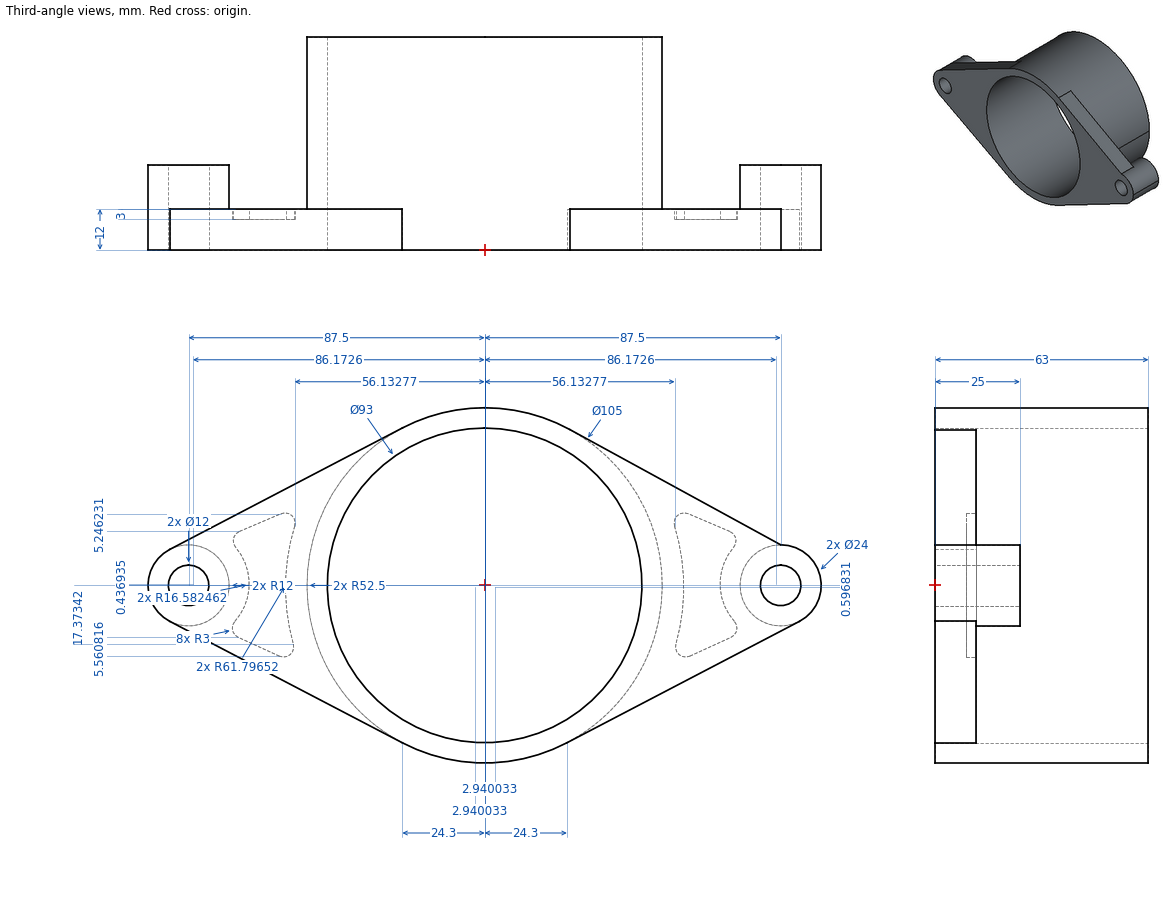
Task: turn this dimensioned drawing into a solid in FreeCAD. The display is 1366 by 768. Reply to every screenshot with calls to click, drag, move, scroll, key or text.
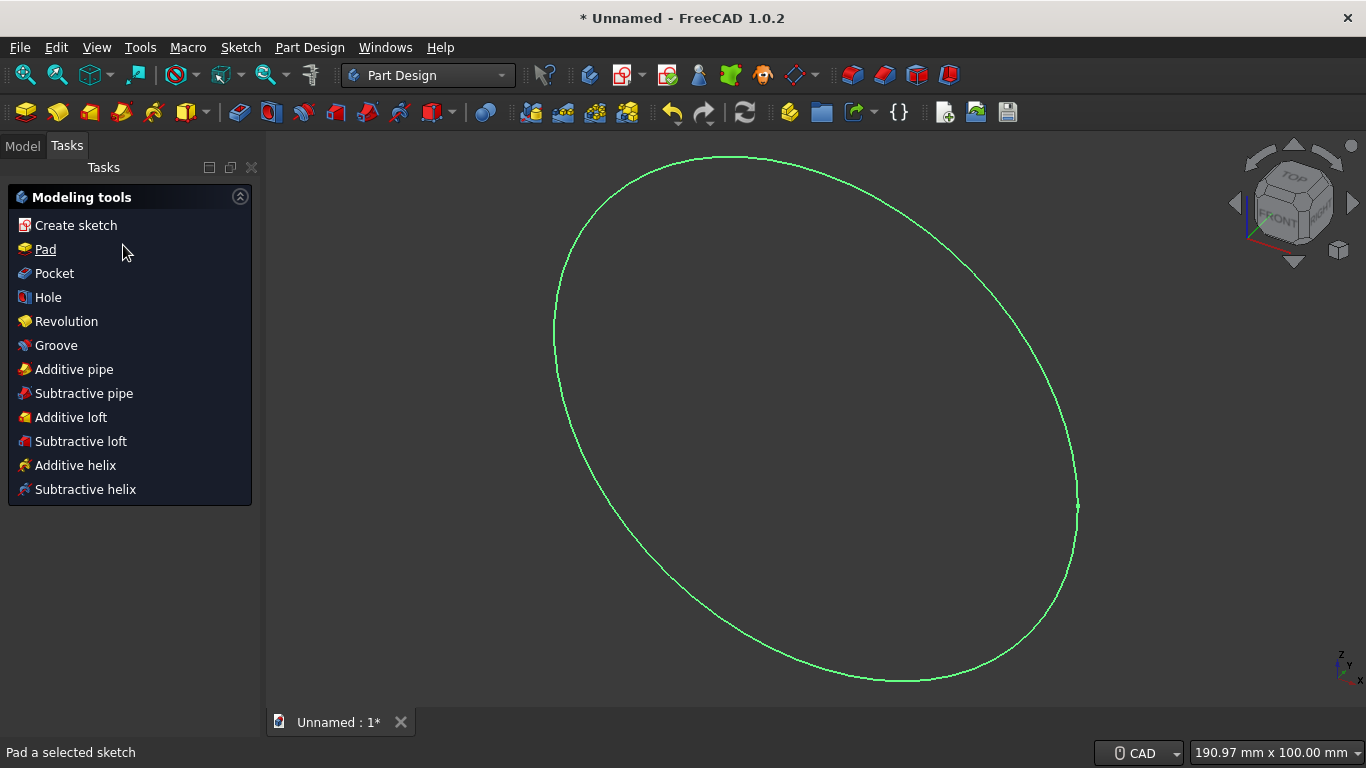
click(26, 112)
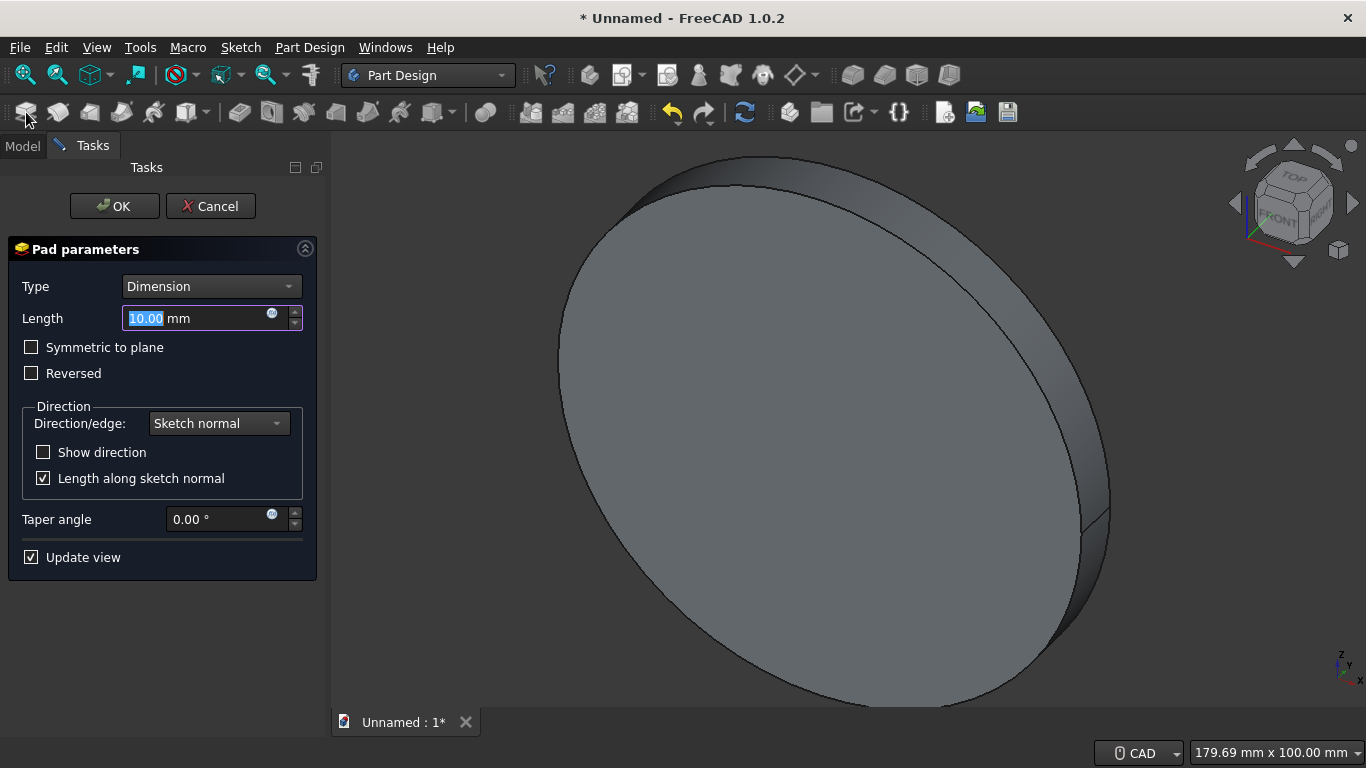
text(63)
key(Tab)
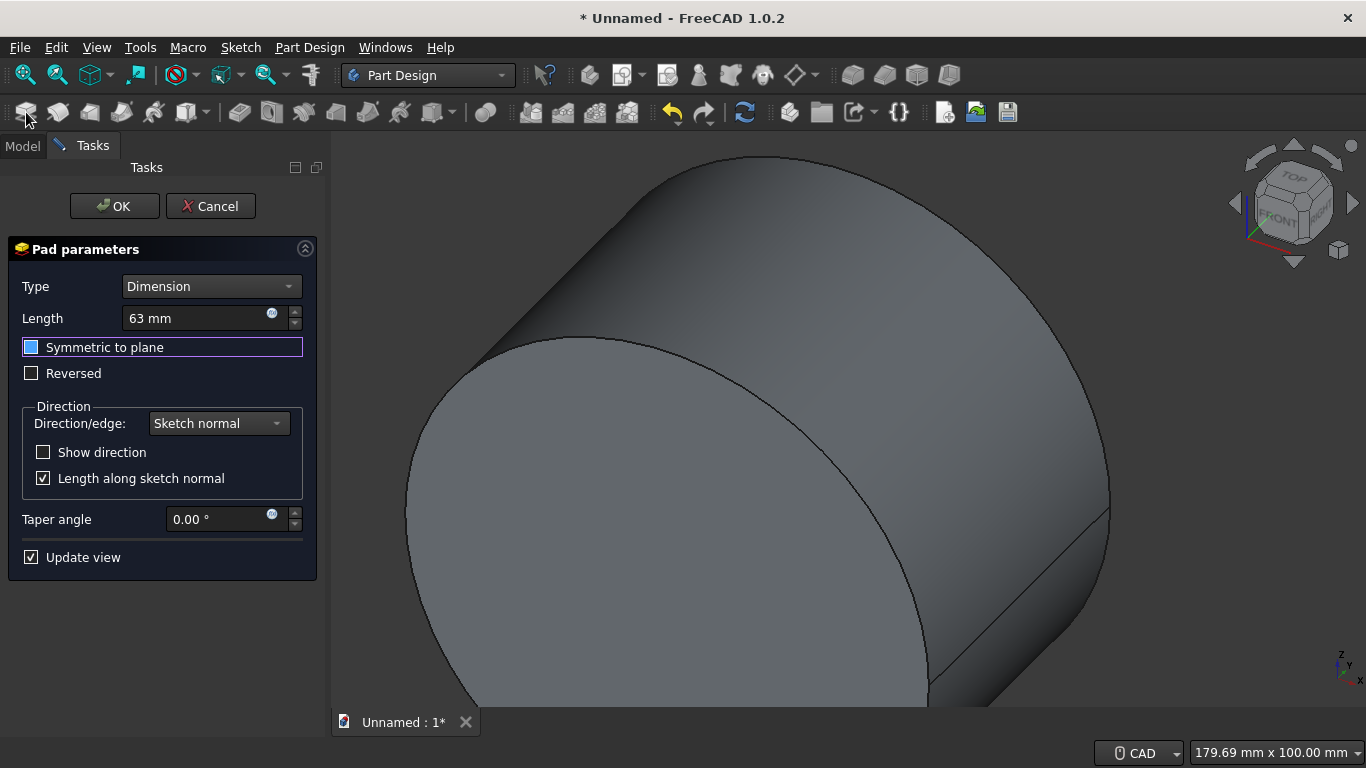
click(30, 373)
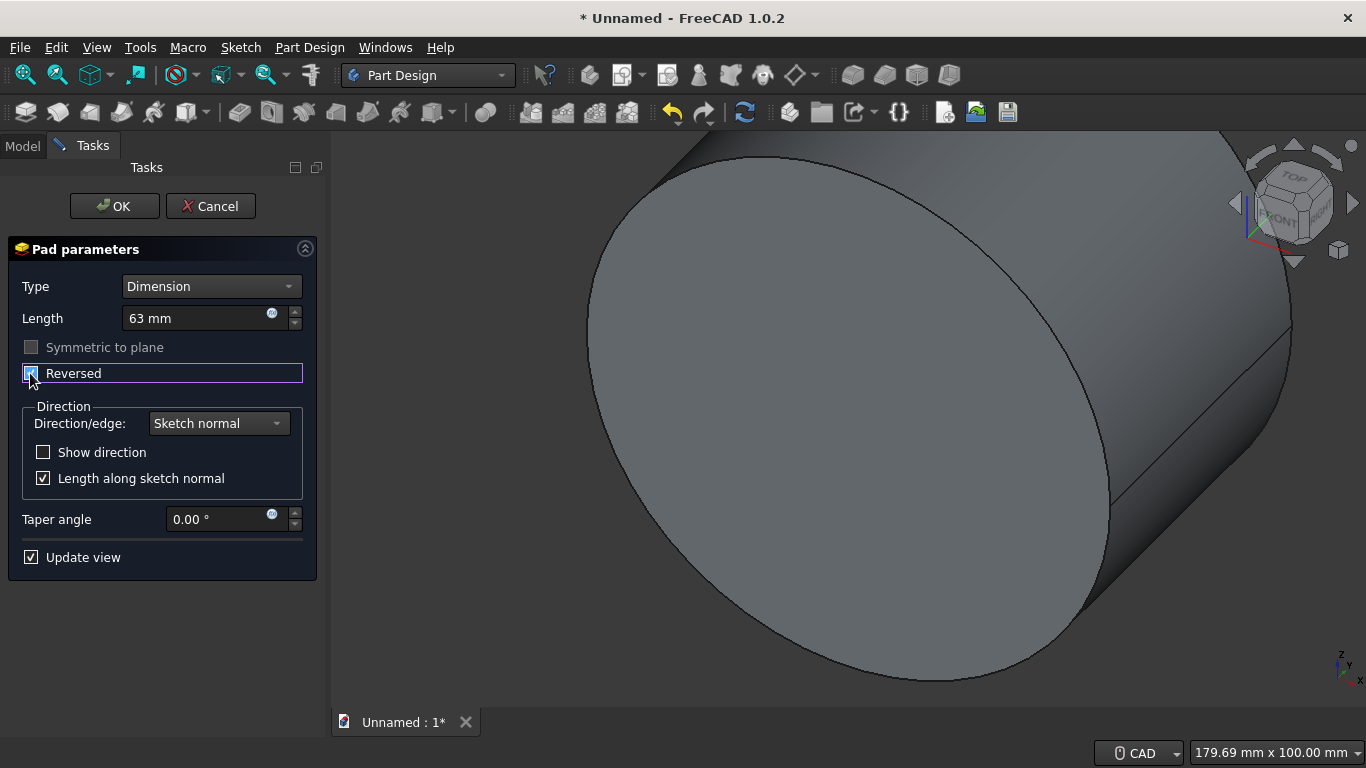
click(115, 206)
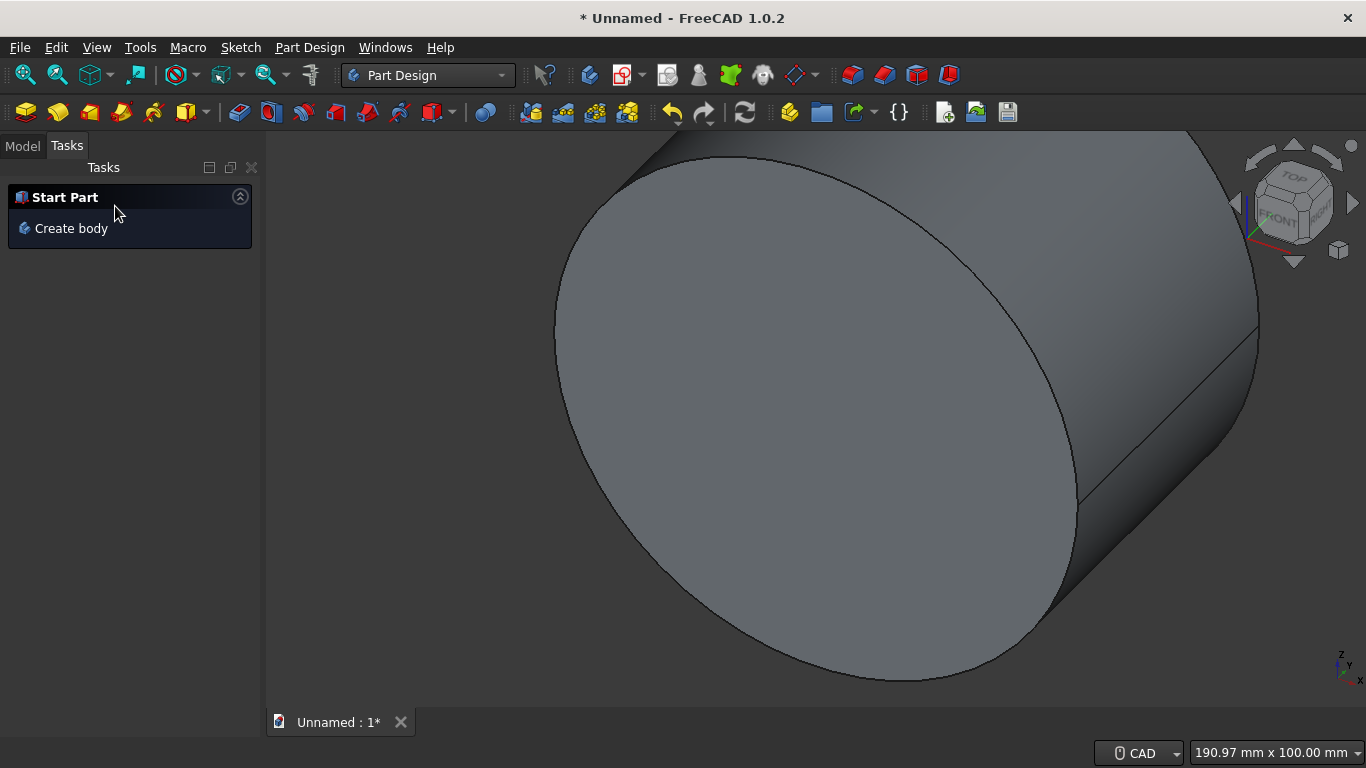
key(v)
key(f)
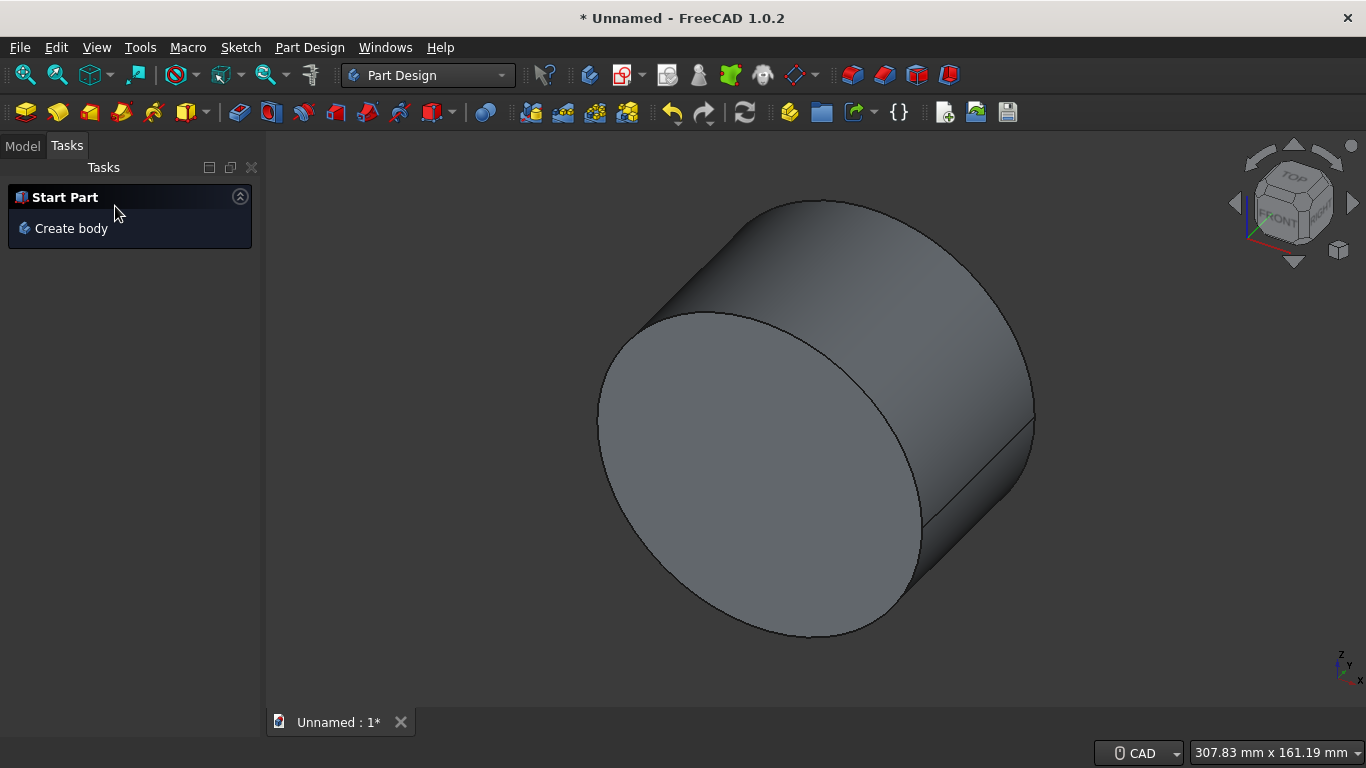
click(760, 474)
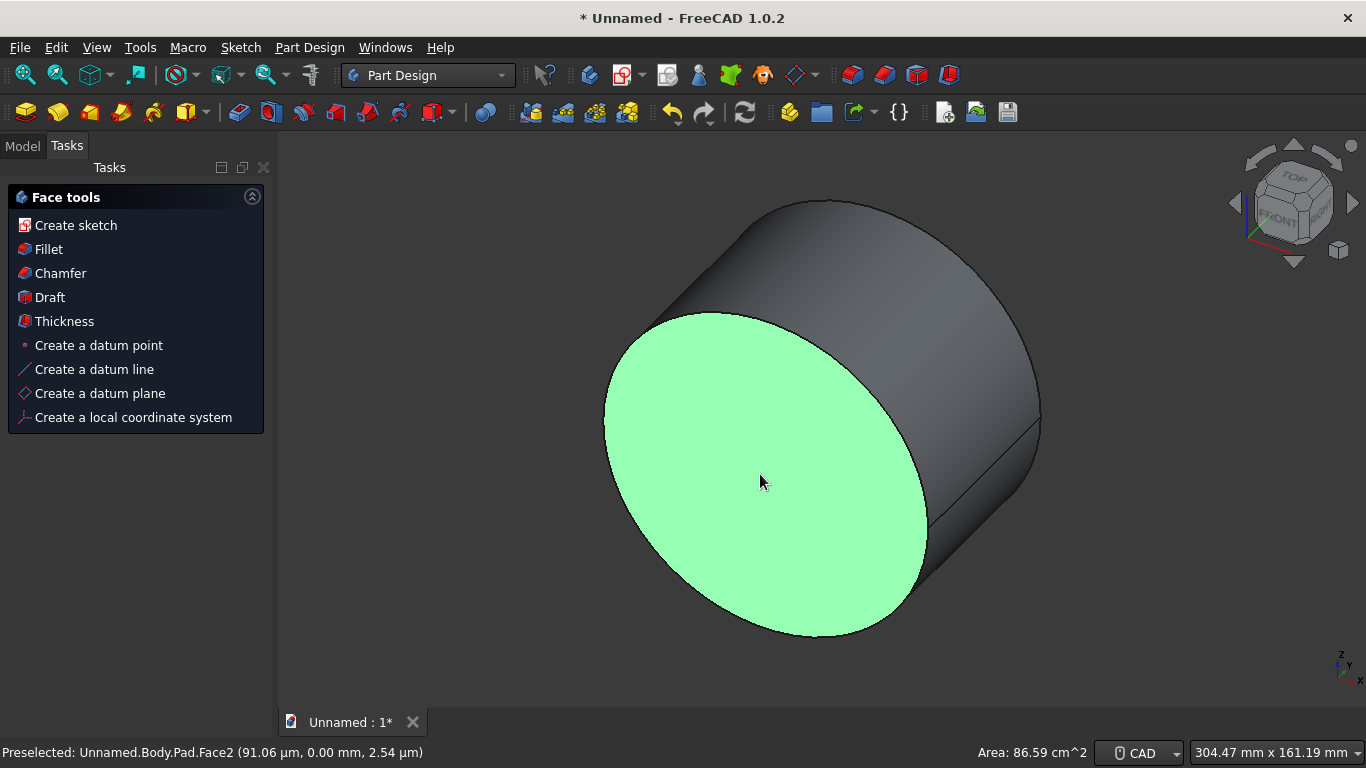
click(622, 76)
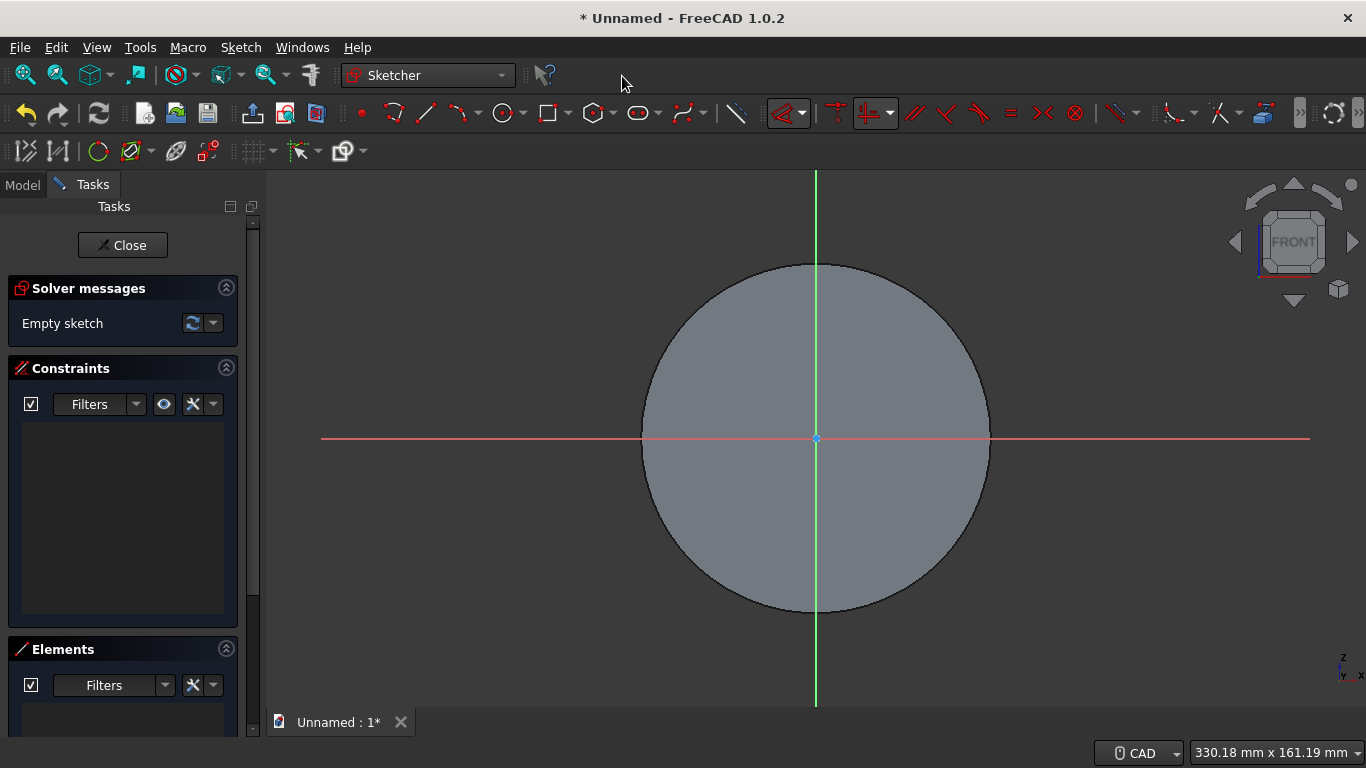
key(g)
key(l)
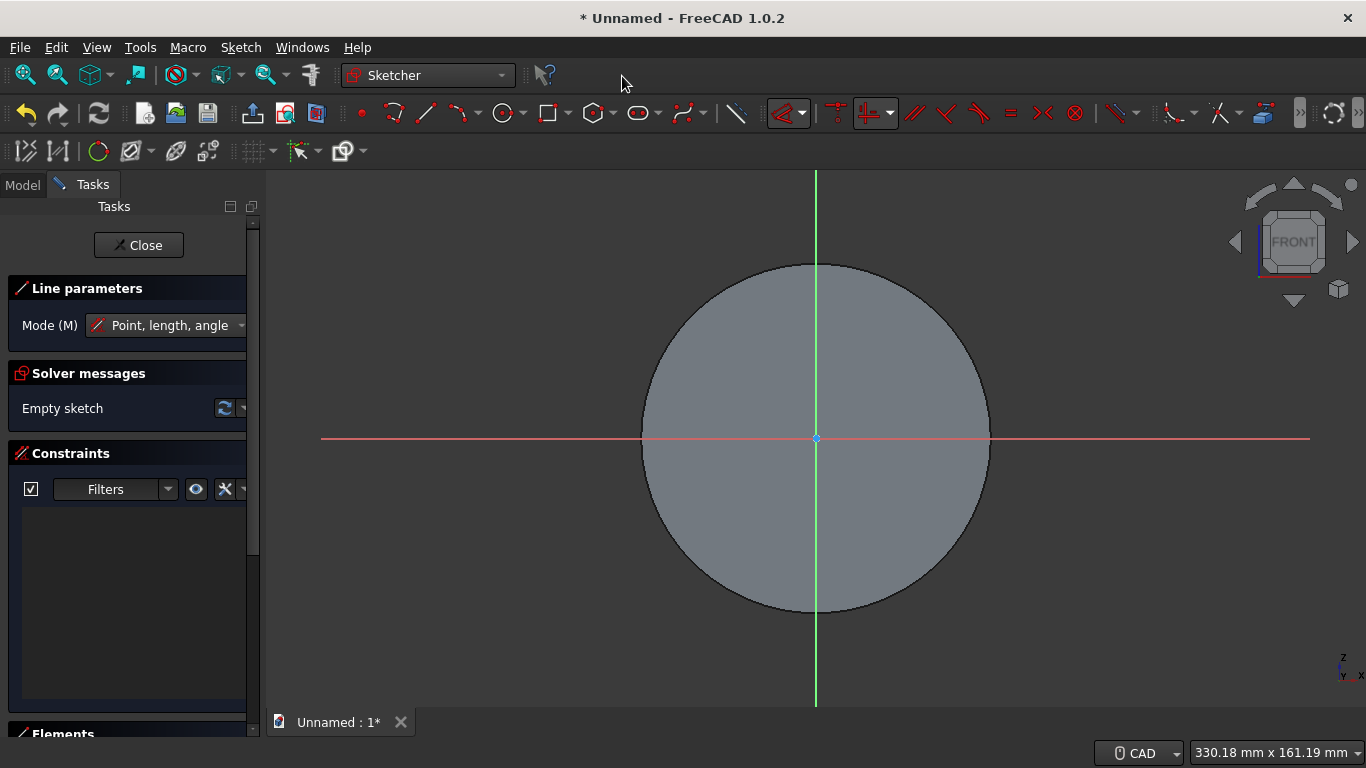
click(735, 594)
click(506, 474)